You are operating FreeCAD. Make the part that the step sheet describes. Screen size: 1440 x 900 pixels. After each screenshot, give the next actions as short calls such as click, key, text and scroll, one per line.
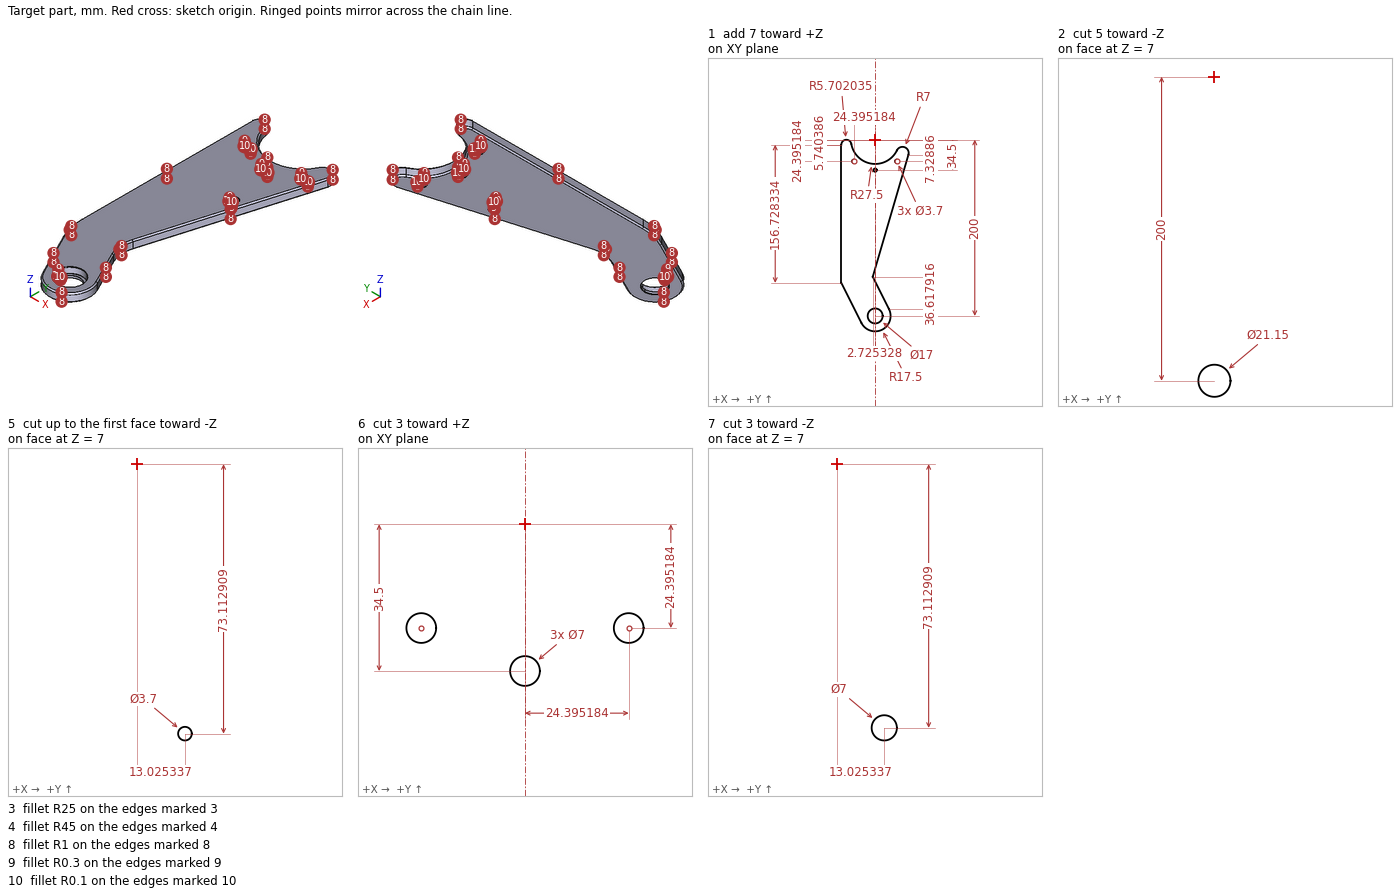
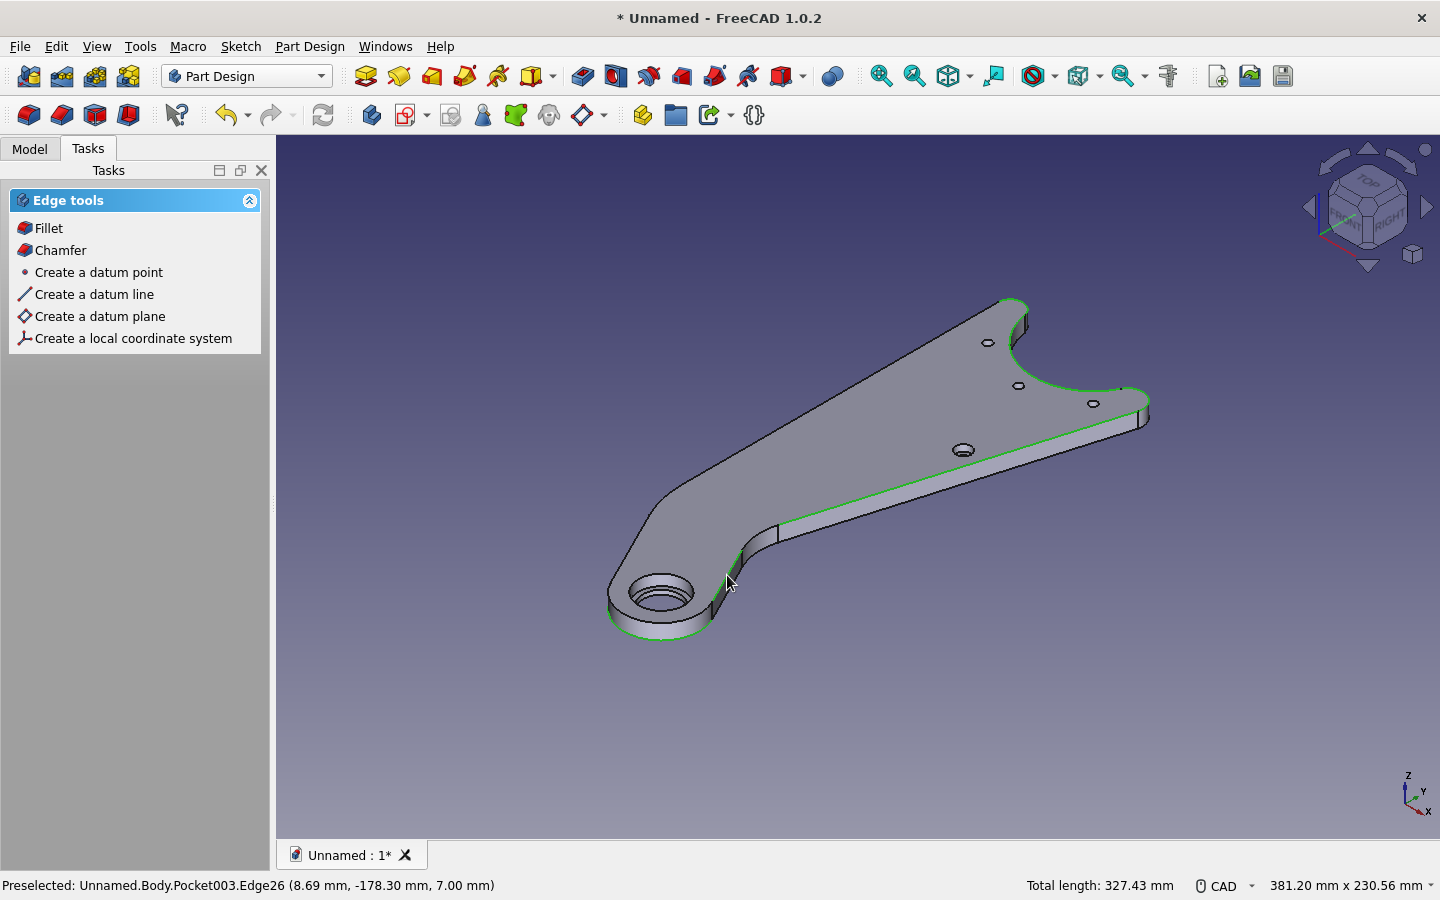
click(756, 535, ctrl)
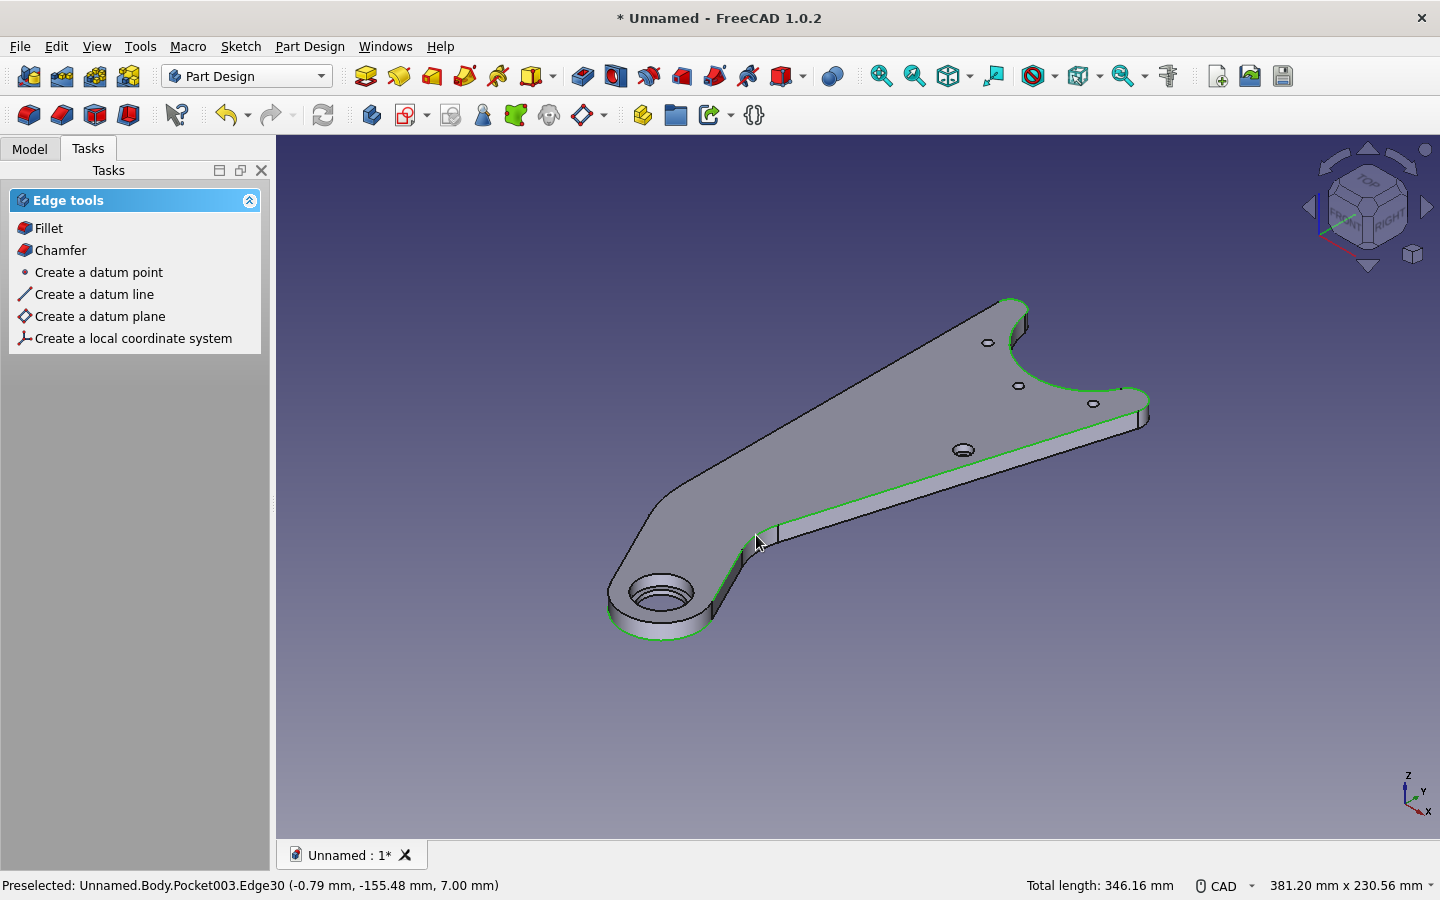
click(674, 489, ctrl)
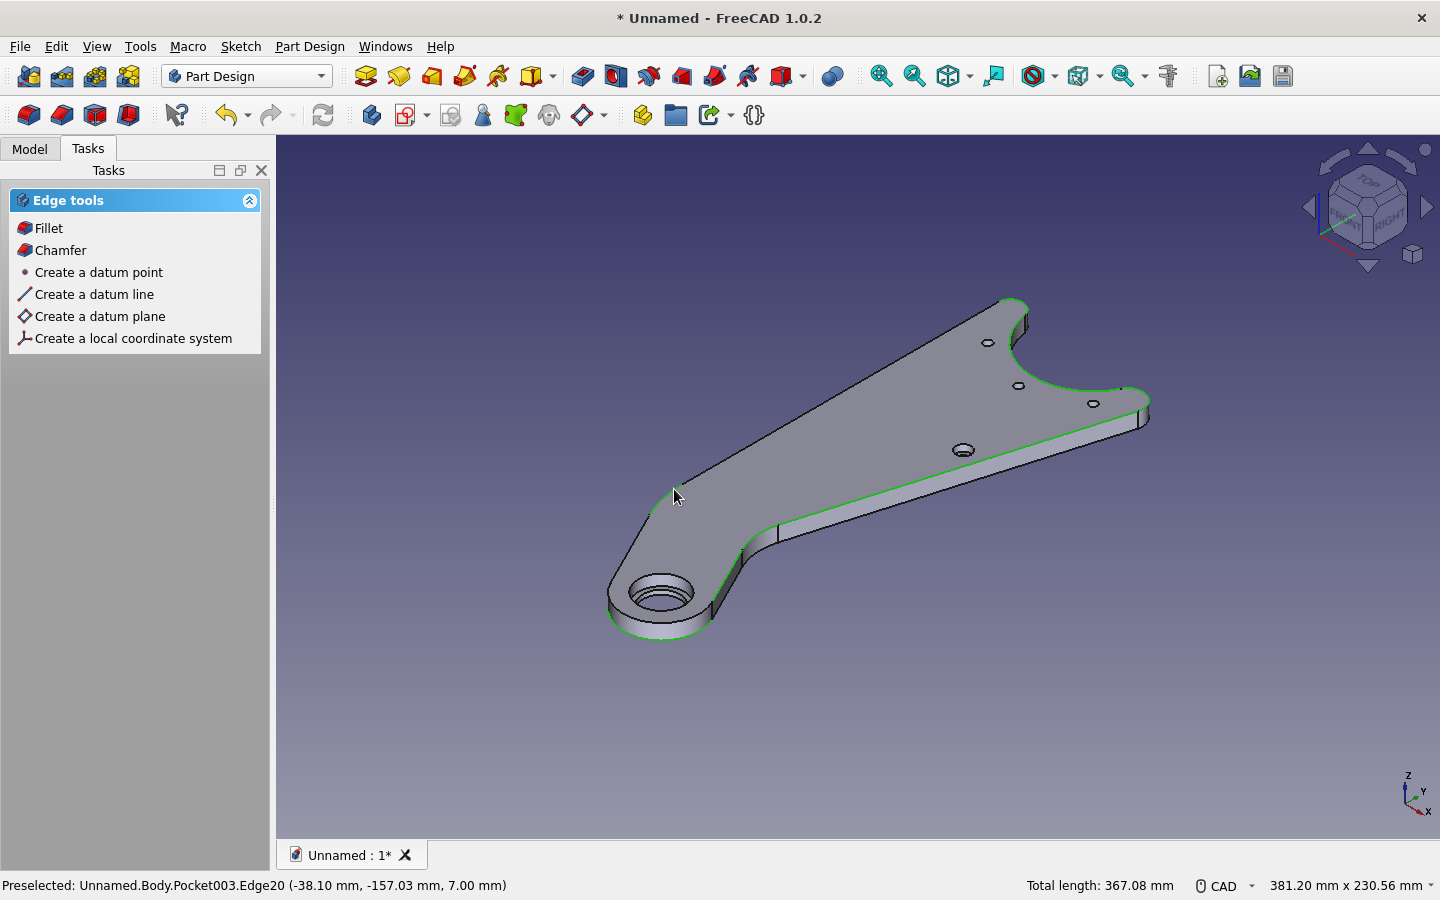
click(645, 621, ctrl)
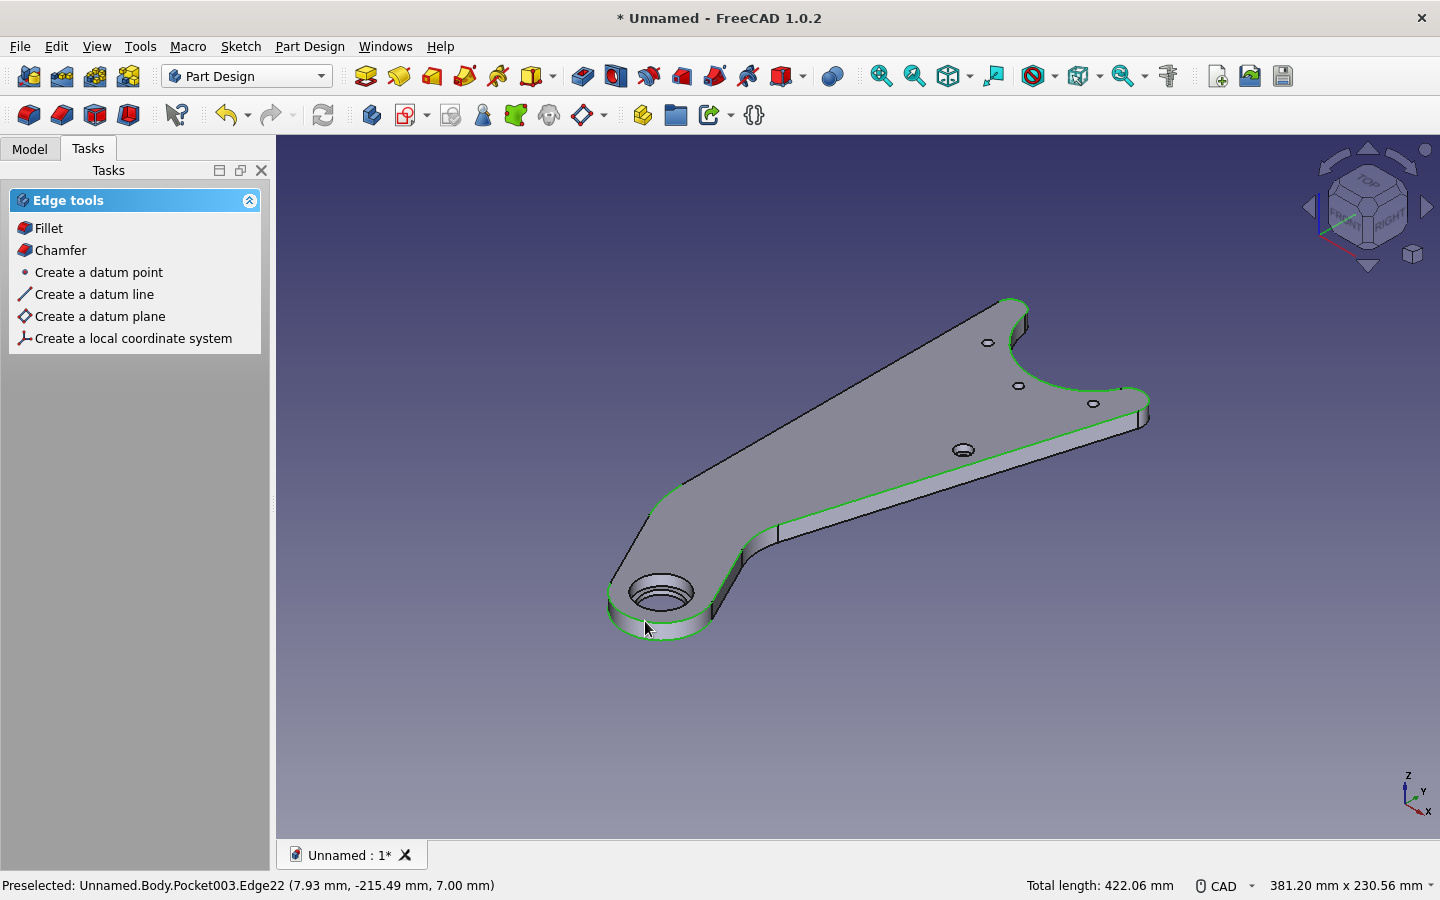
key(2)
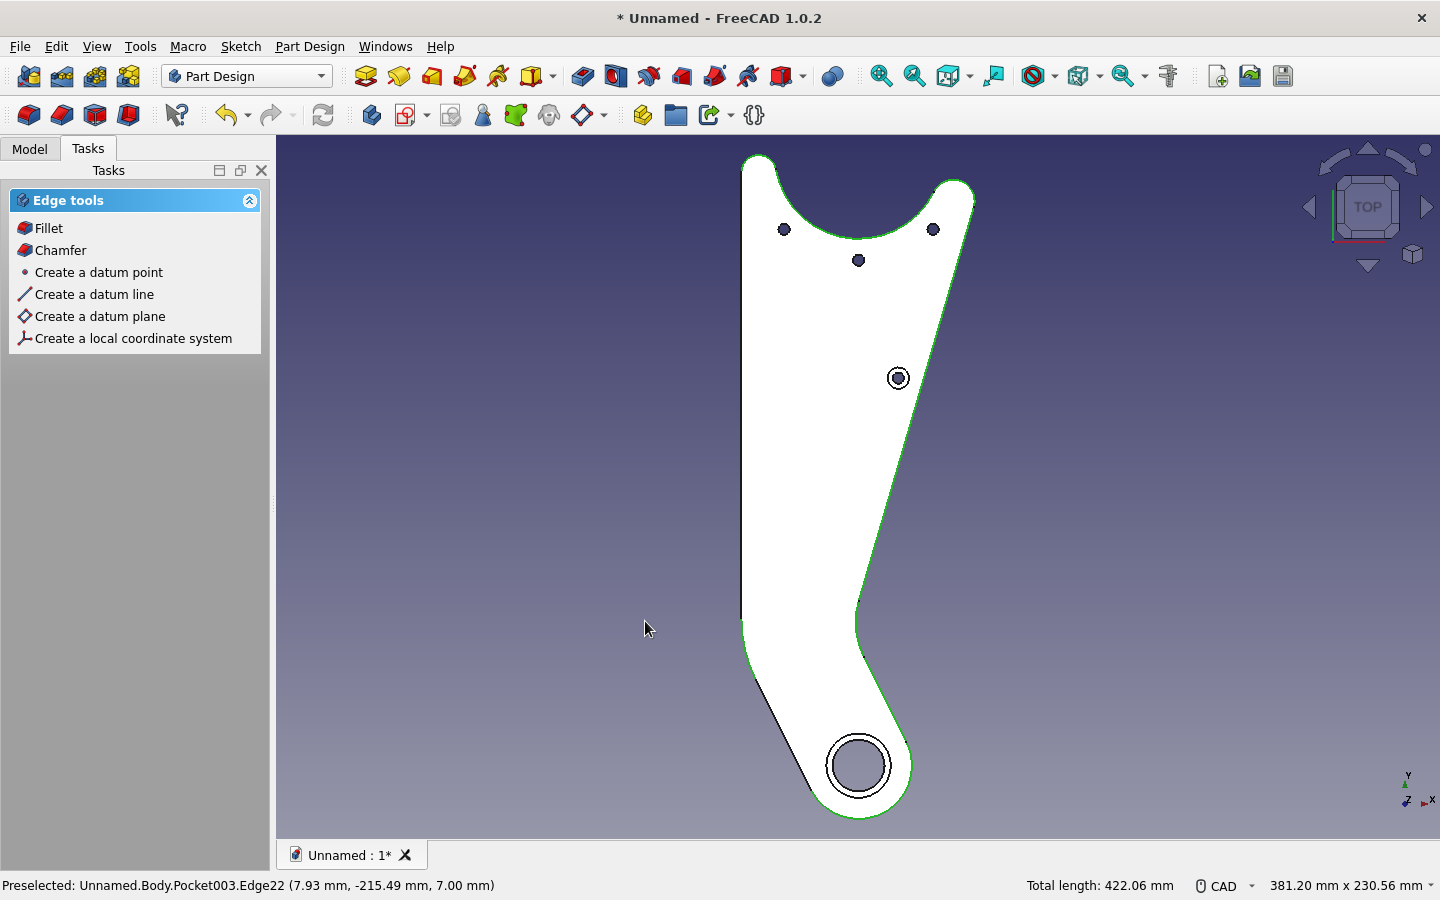
click(741, 394, ctrl)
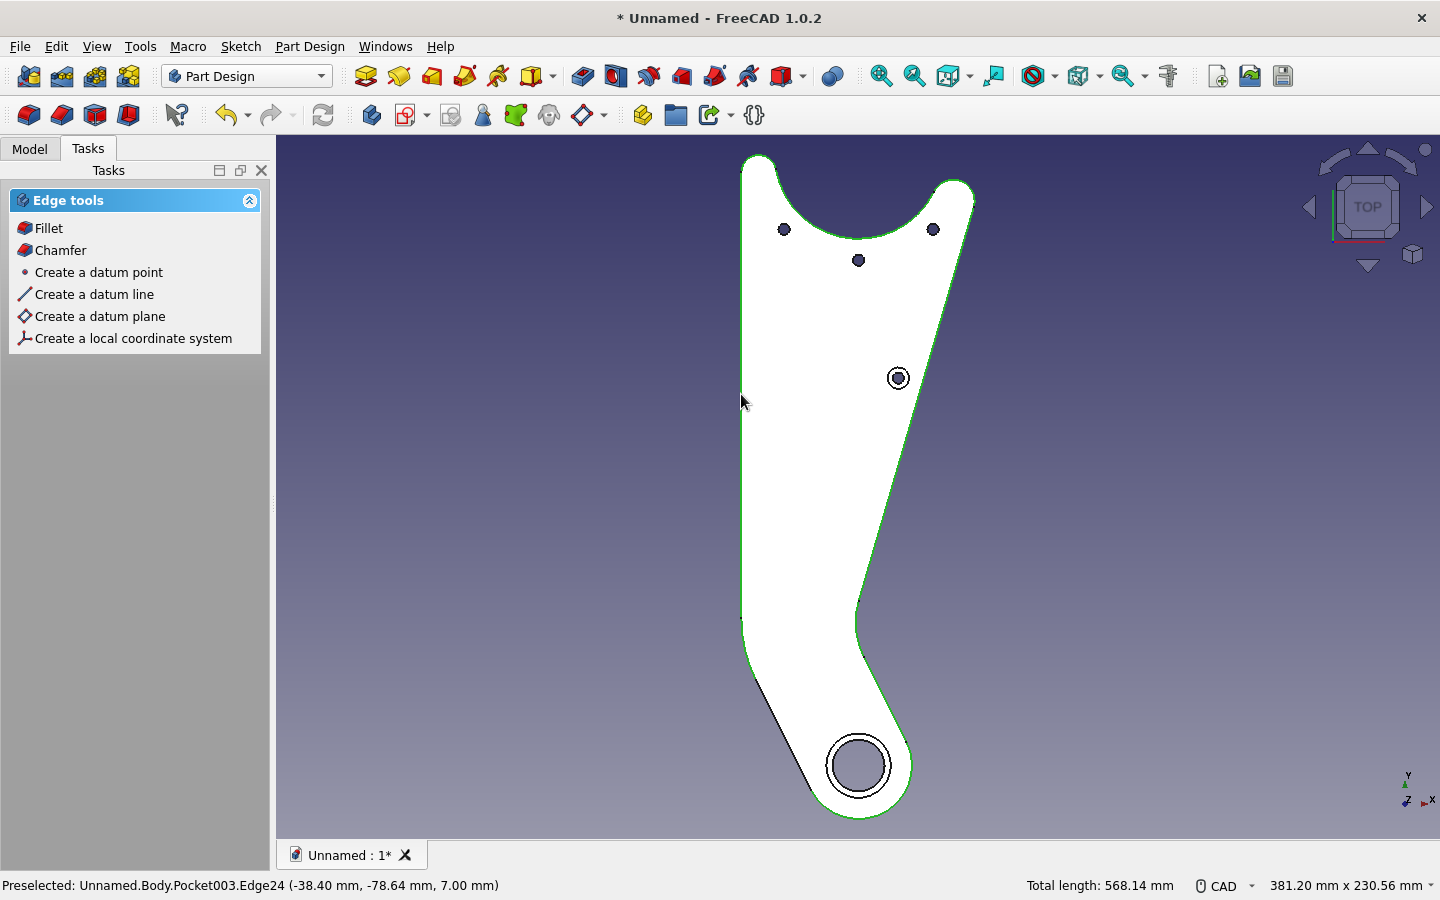
click(783, 734, ctrl)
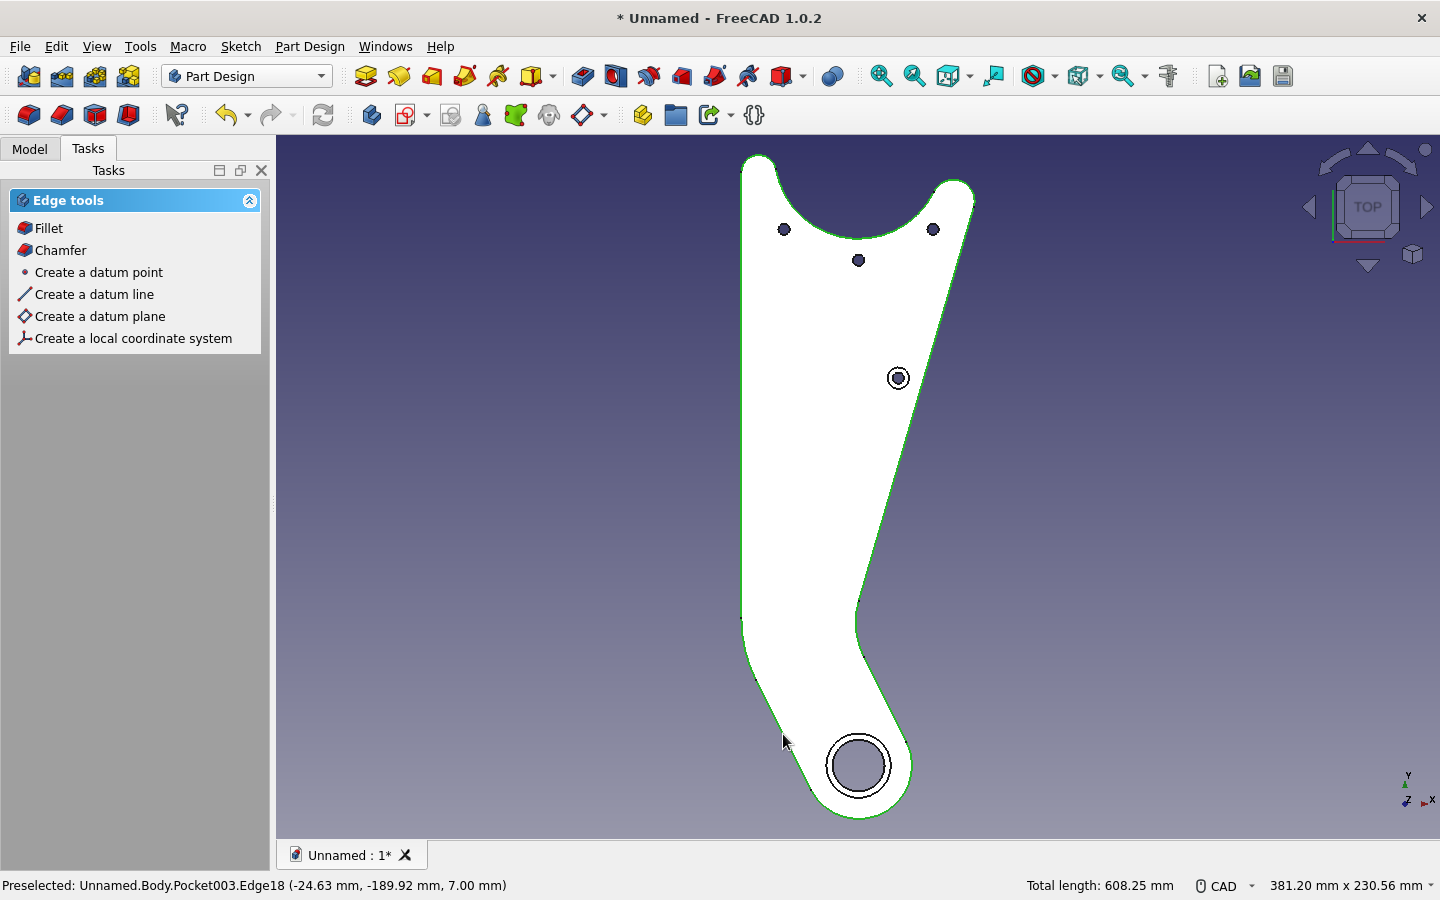
key(0)